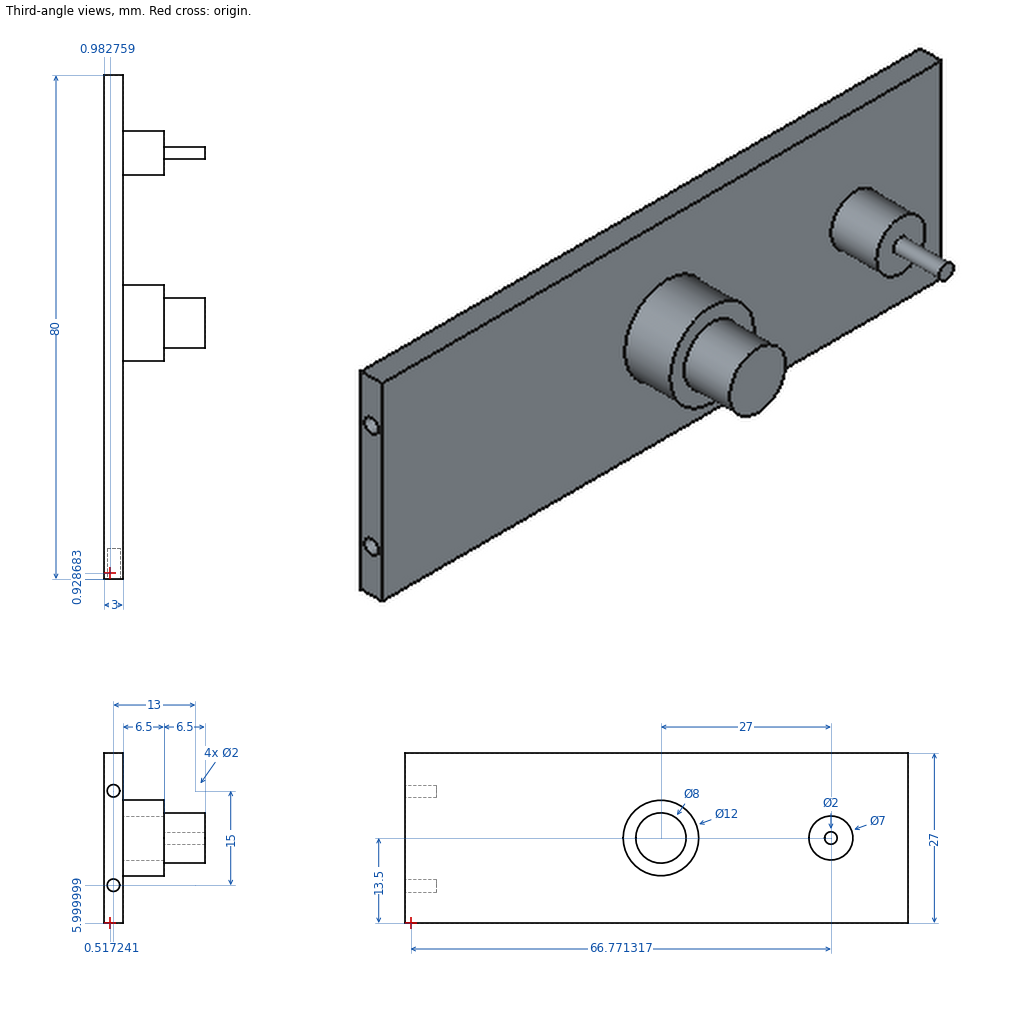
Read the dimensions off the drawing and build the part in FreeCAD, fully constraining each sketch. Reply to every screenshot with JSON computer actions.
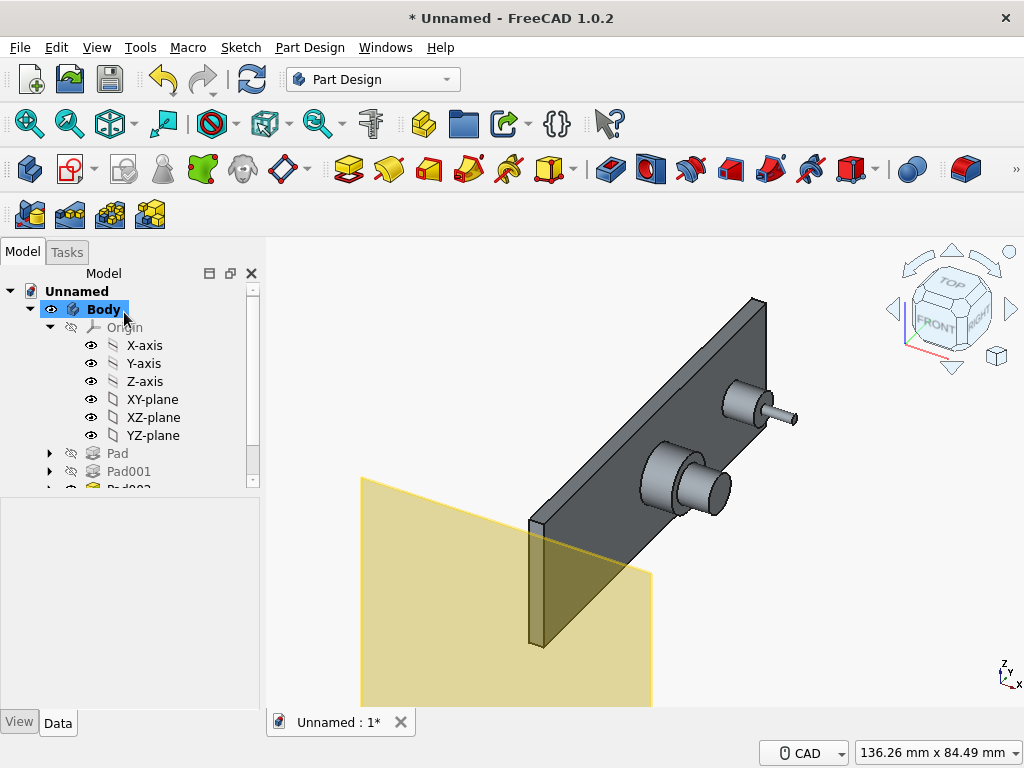
{"action": "scroll", "coordinate": [100, 377], "scroll_direction": "down", "scroll_amount": 3}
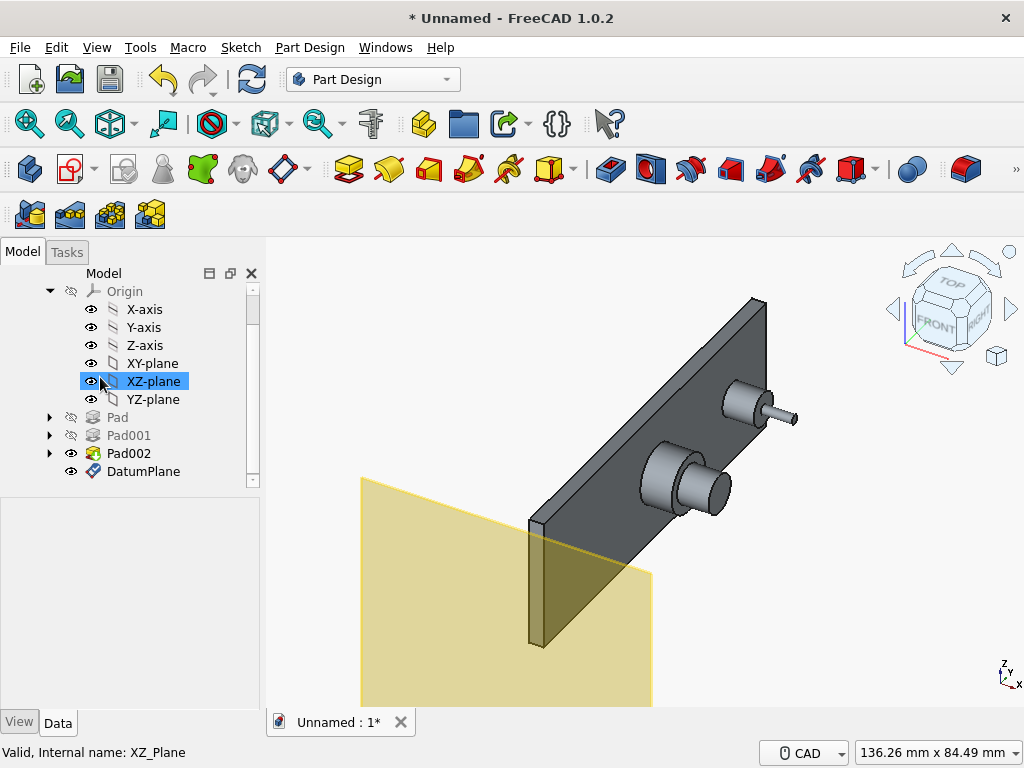
{"action": "left_click", "coordinate": [116, 471]}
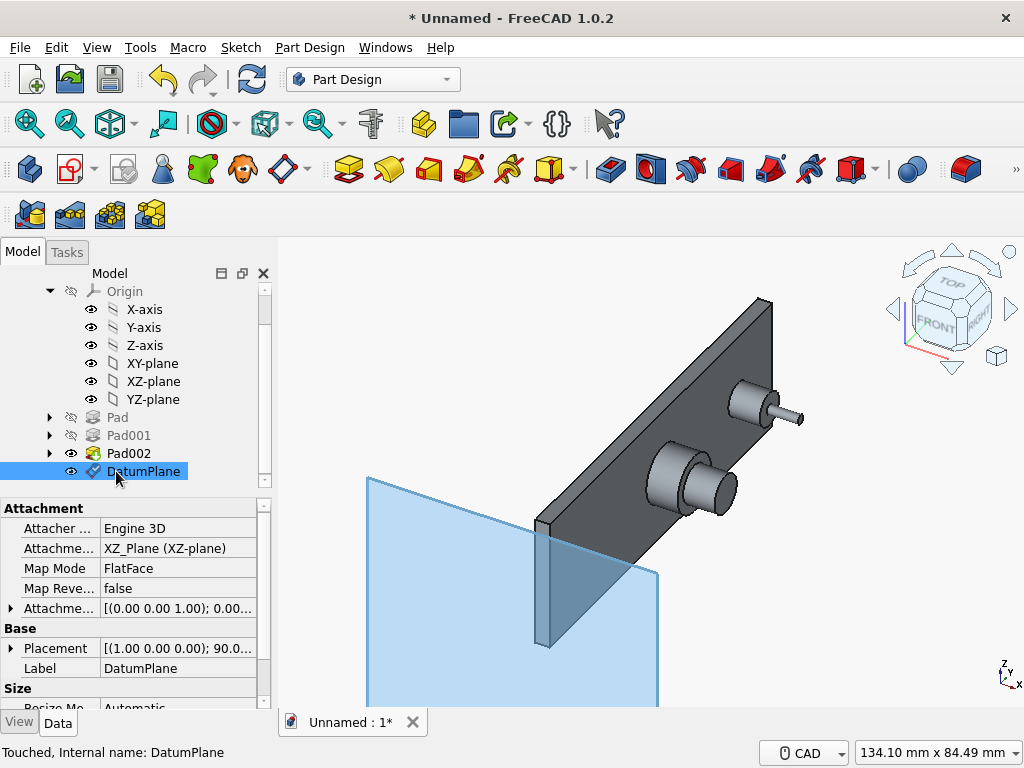
{"action": "left_click", "coordinate": [70, 170]}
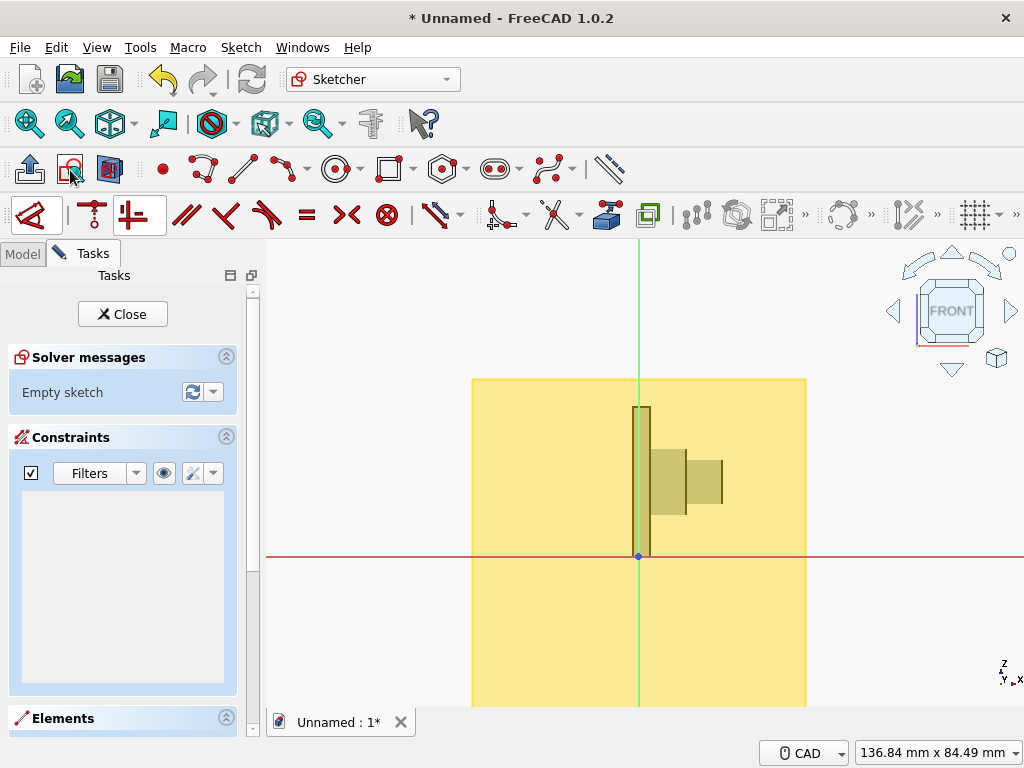
{"action": "scroll", "coordinate": [760, 515], "scroll_direction": "up", "scroll_amount": 4}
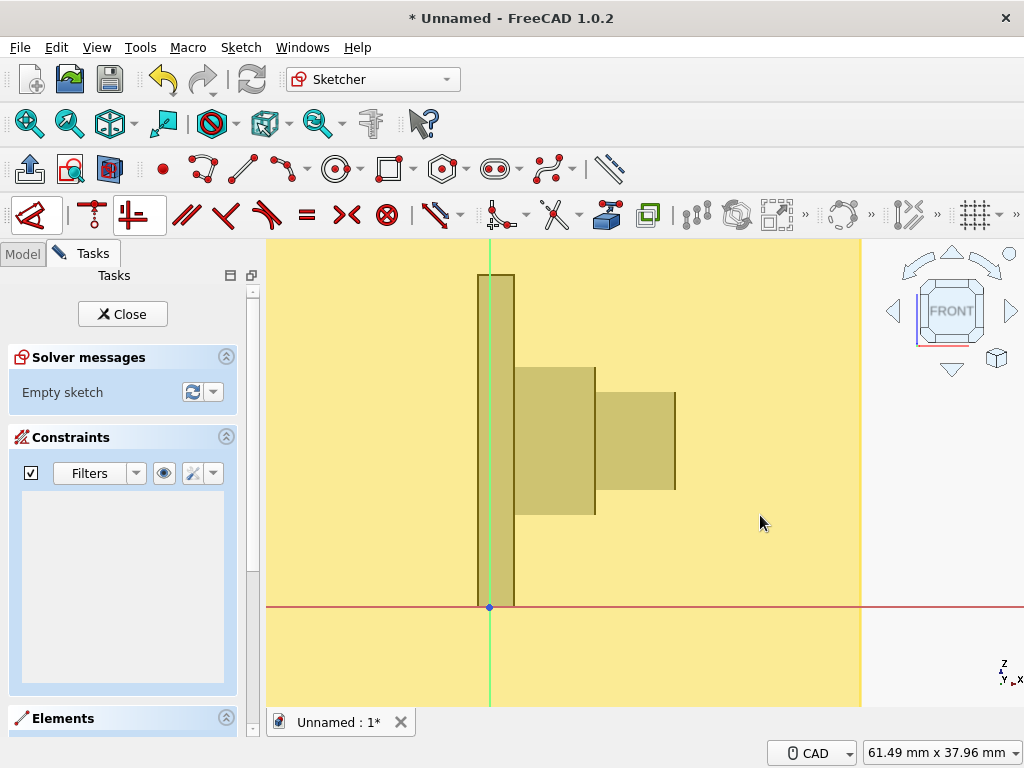
{"action": "left_click", "coordinate": [336, 170]}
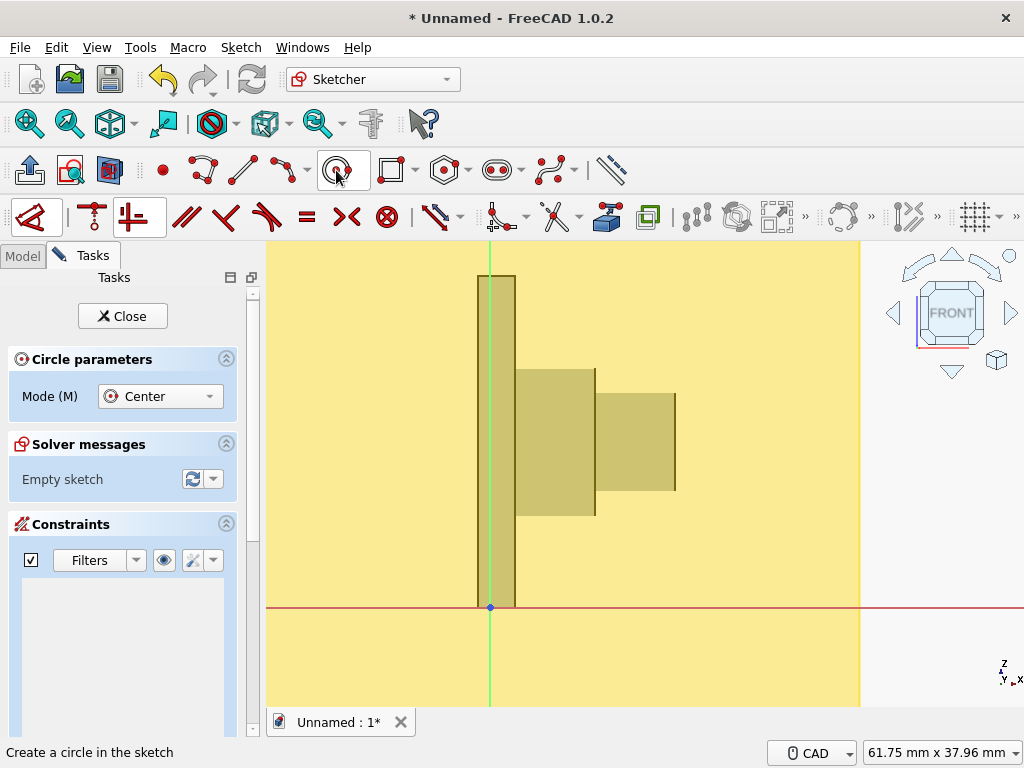
{"action": "scroll", "coordinate": [656, 350], "scroll_direction": "up", "scroll_amount": 4}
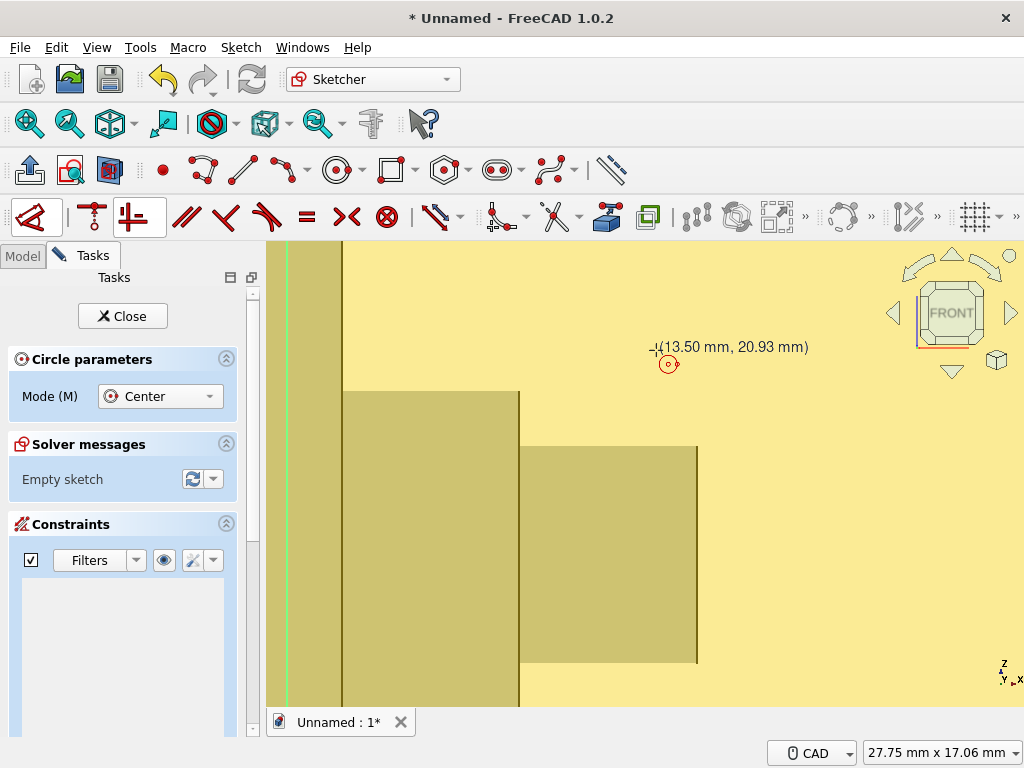
{"action": "left_click", "coordinate": [656, 350]}
{"action": "mouse_move", "coordinate": [675, 331]}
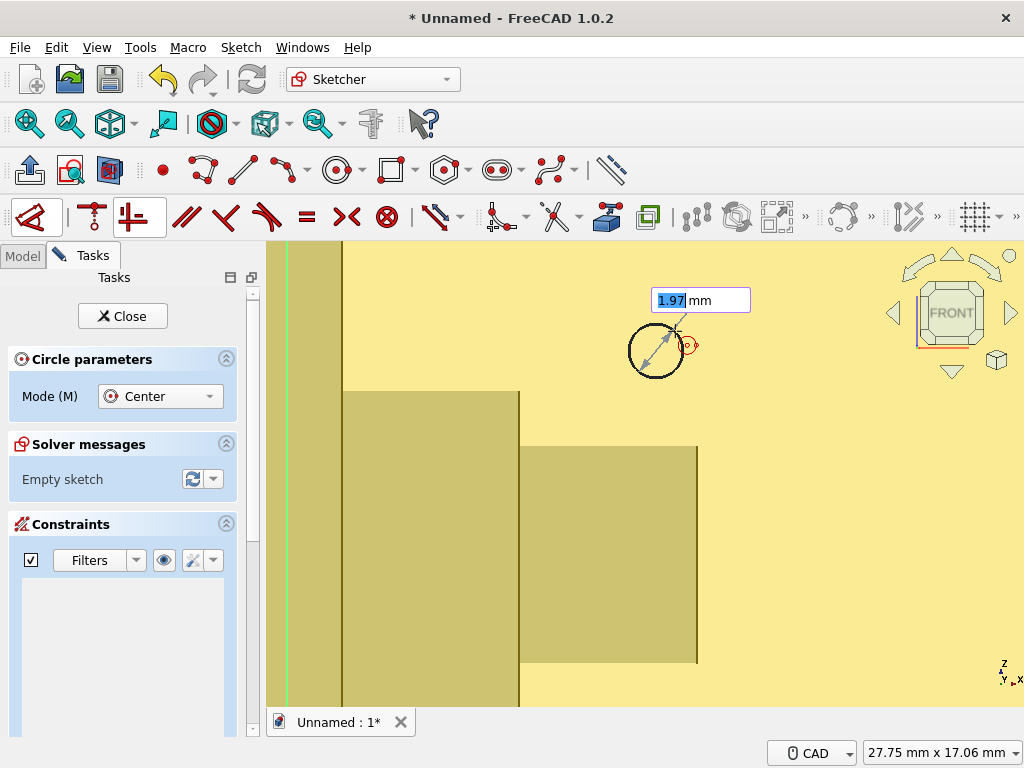
{"action": "type", "text": "2"}
{"action": "key", "text": "Return"}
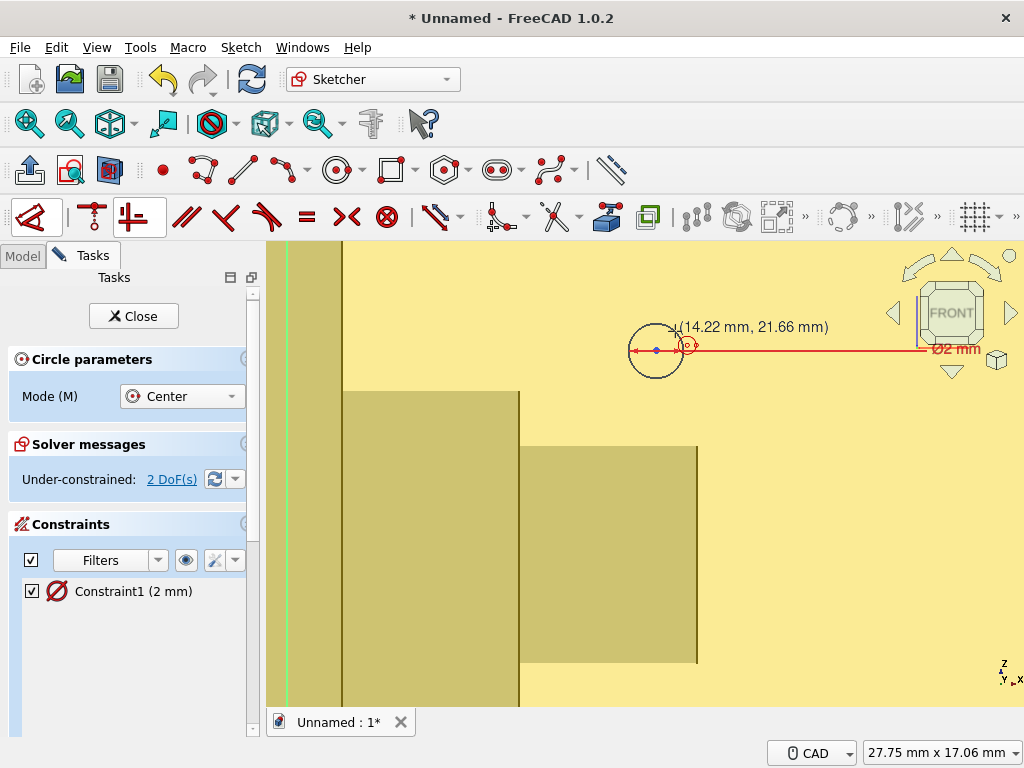
{"action": "scroll", "coordinate": [657, 352], "scroll_direction": "down", "scroll_amount": 4}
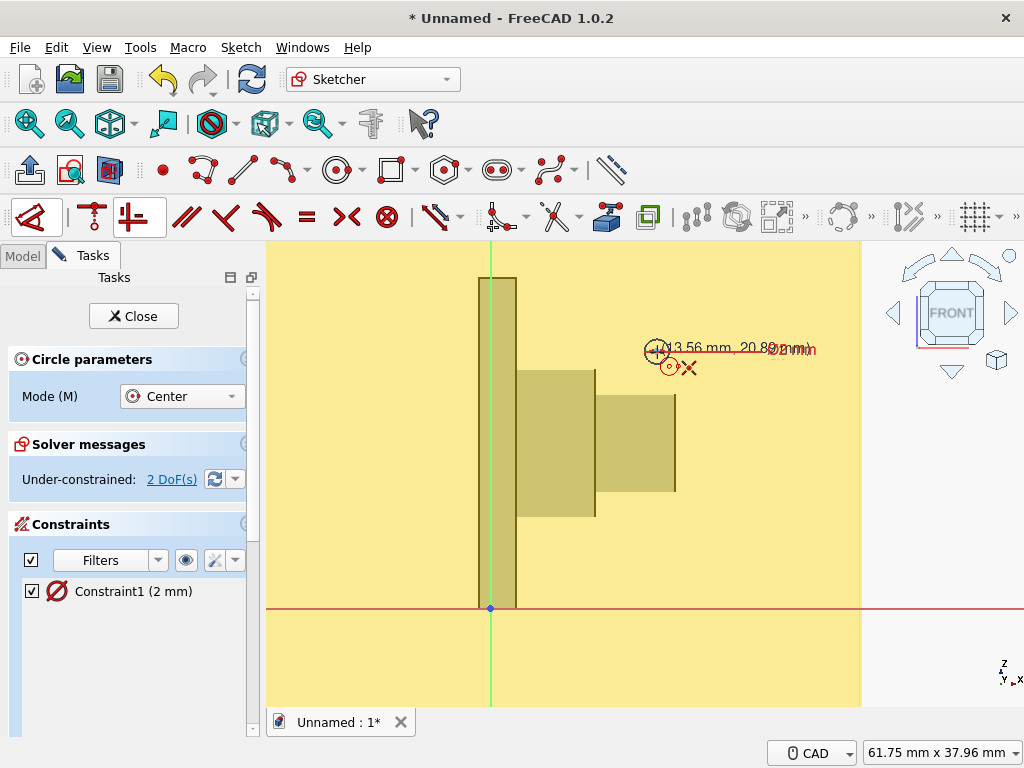
{"action": "scroll", "coordinate": [657, 535], "scroll_direction": "up", "scroll_amount": 4}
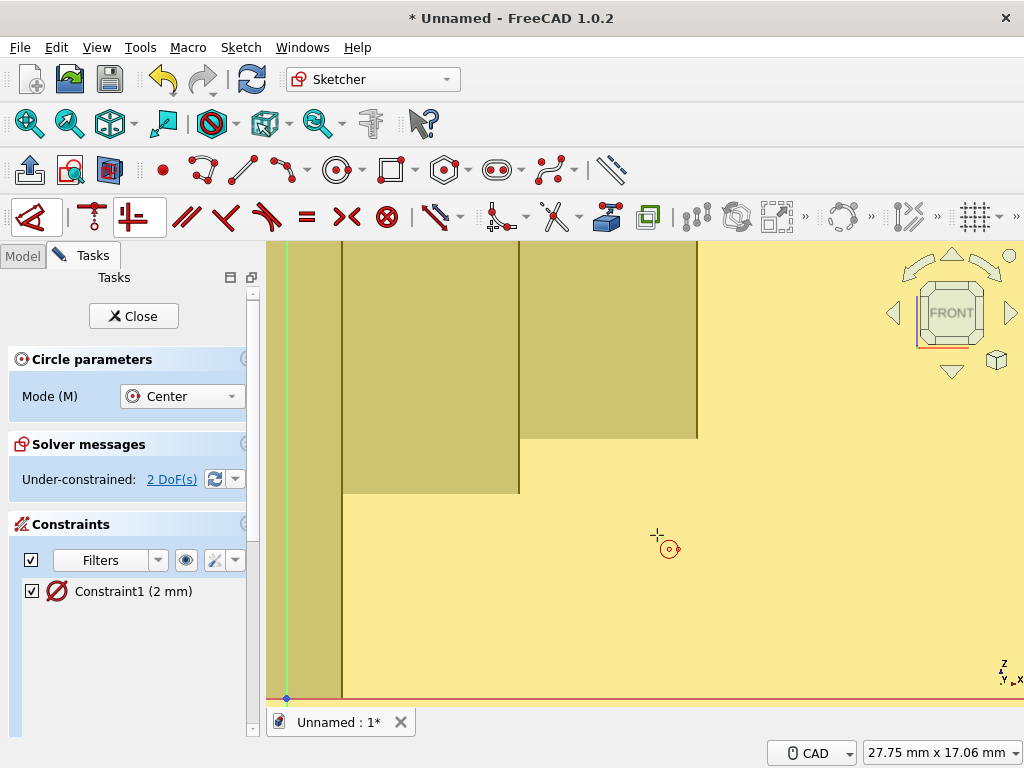
{"action": "left_click", "coordinate": [656, 535]}
{"action": "mouse_move", "coordinate": [675, 516]}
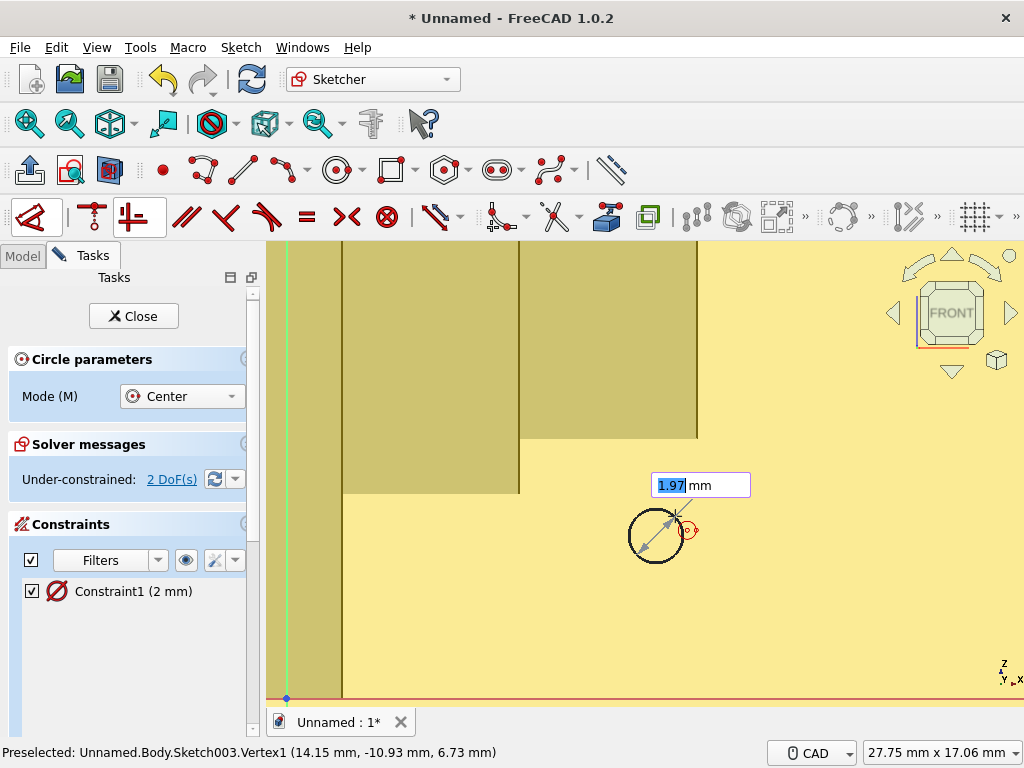
{"action": "type", "text": "2"}
{"action": "key", "text": "Return"}